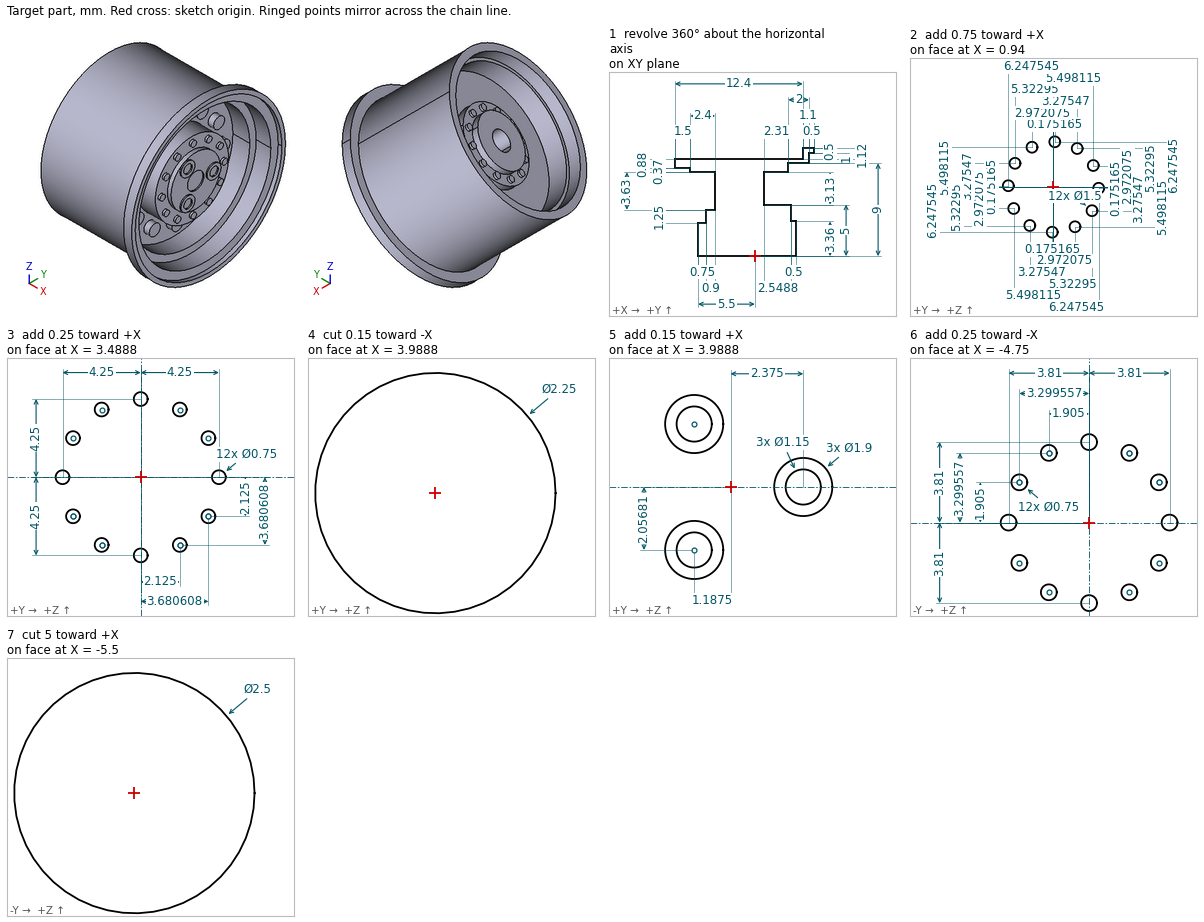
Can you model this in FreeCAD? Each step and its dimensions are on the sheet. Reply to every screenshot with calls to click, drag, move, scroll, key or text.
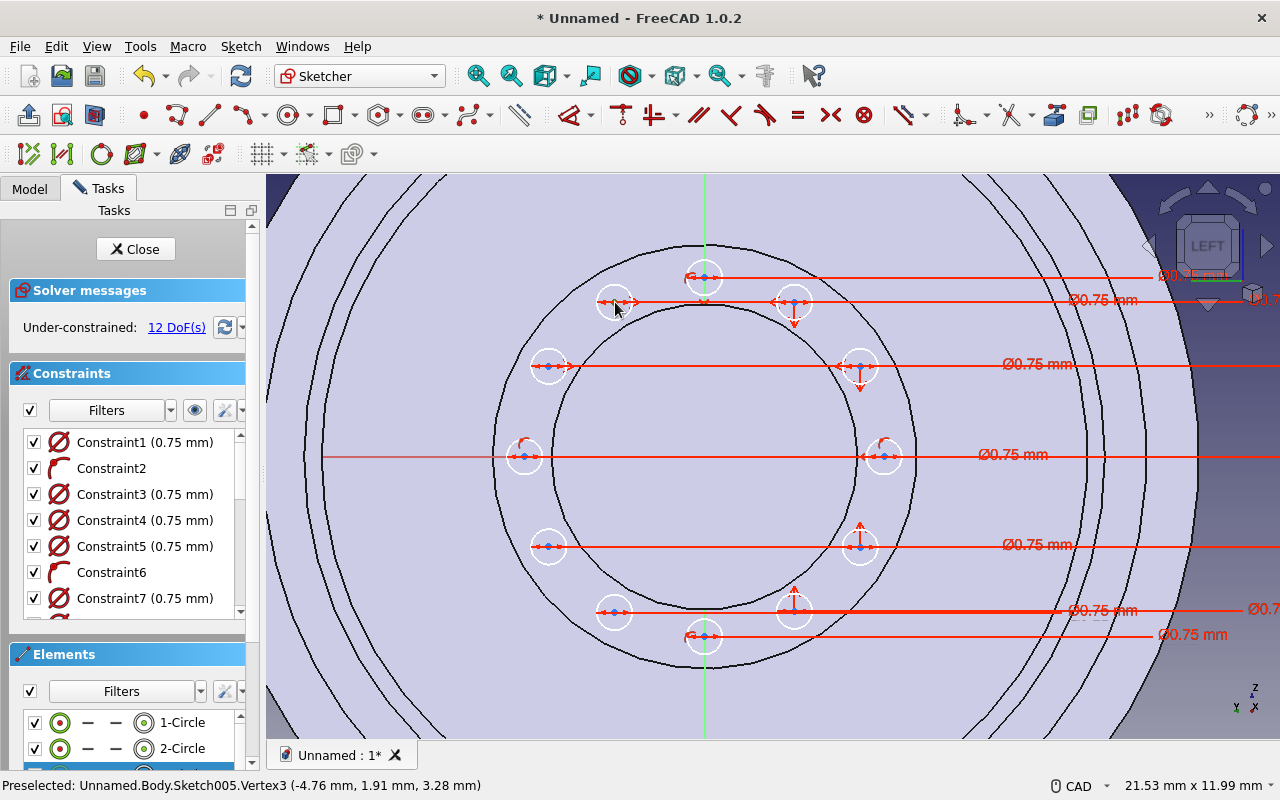
click(615, 613)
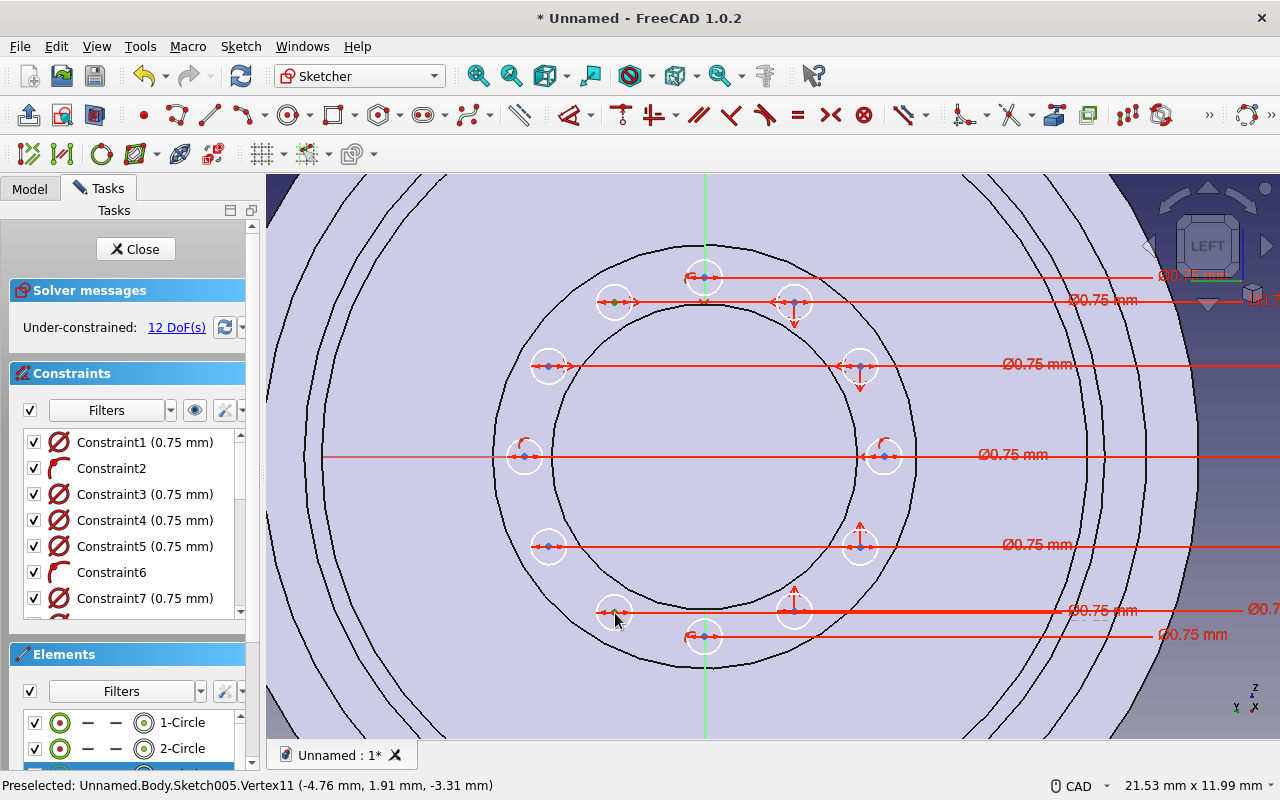
click(353, 457)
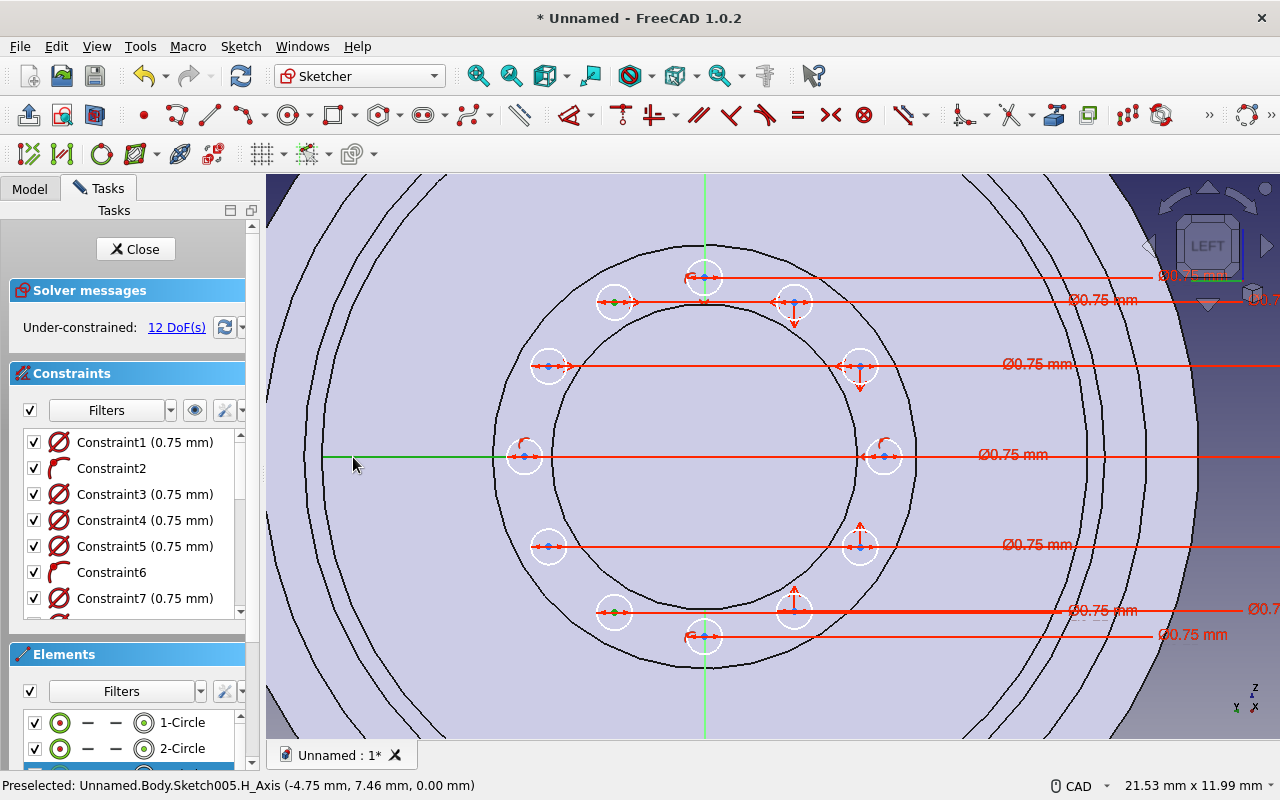
click(831, 116)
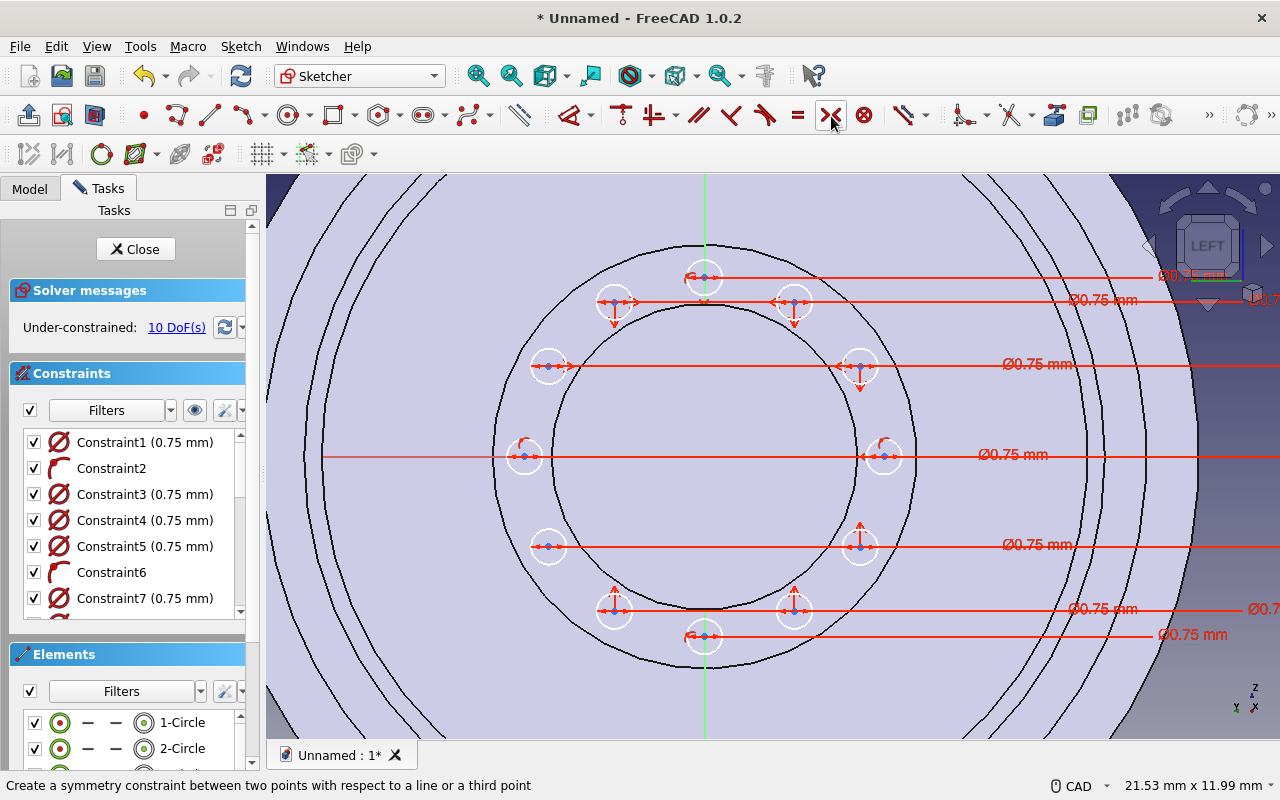
click(549, 366)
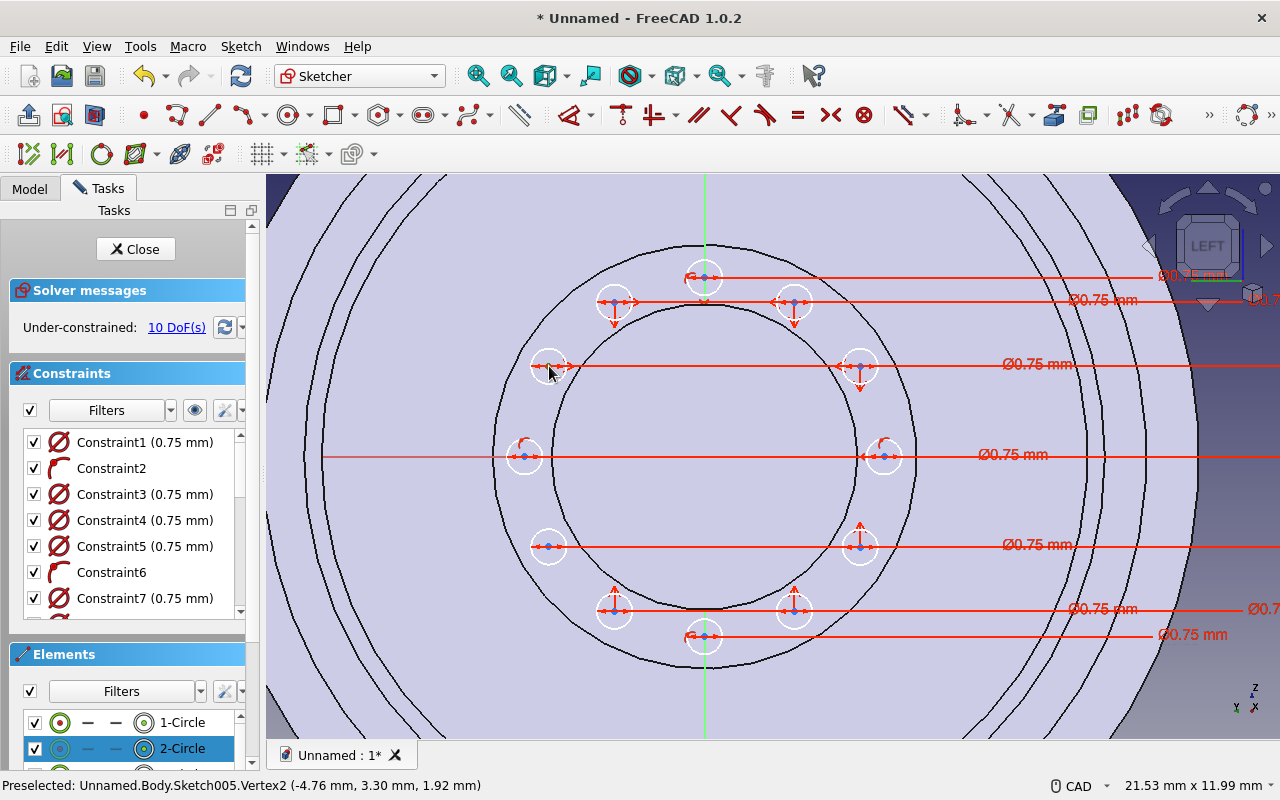
click(549, 547)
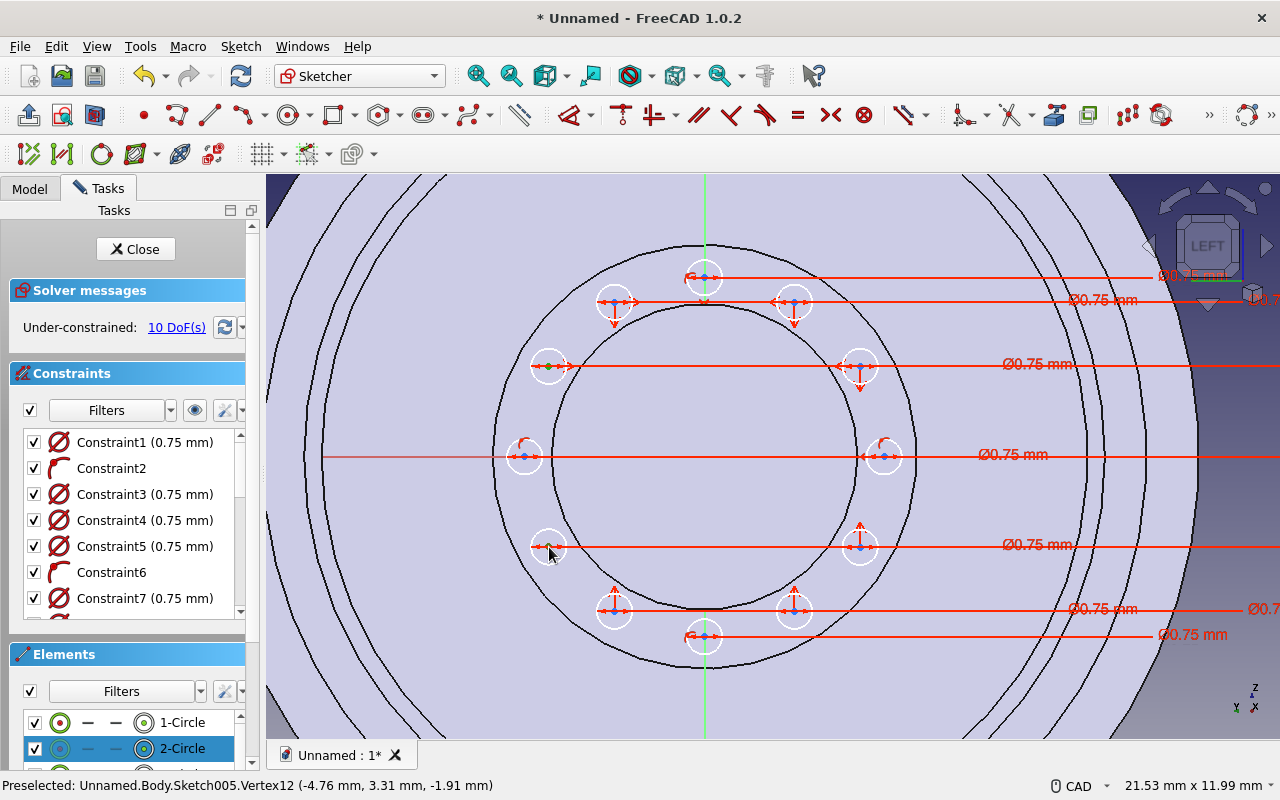
click(353, 457)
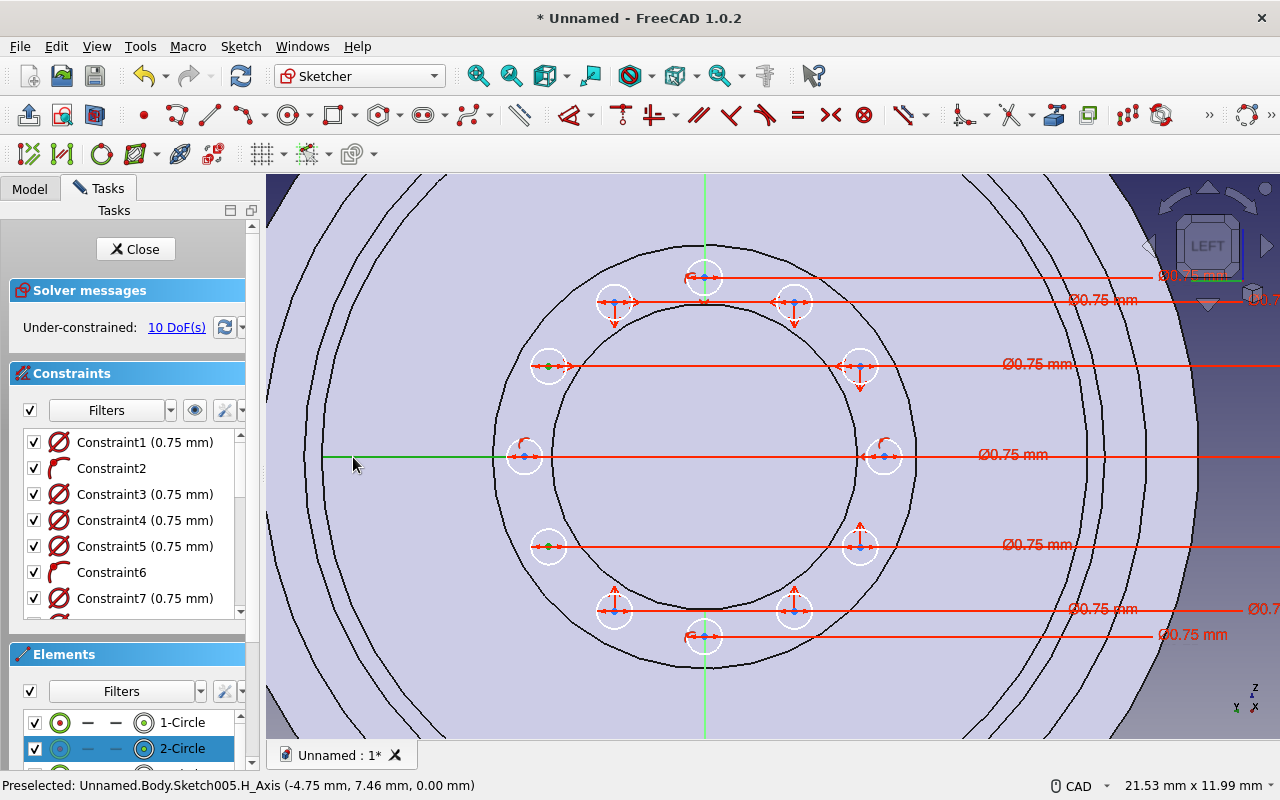
click(831, 116)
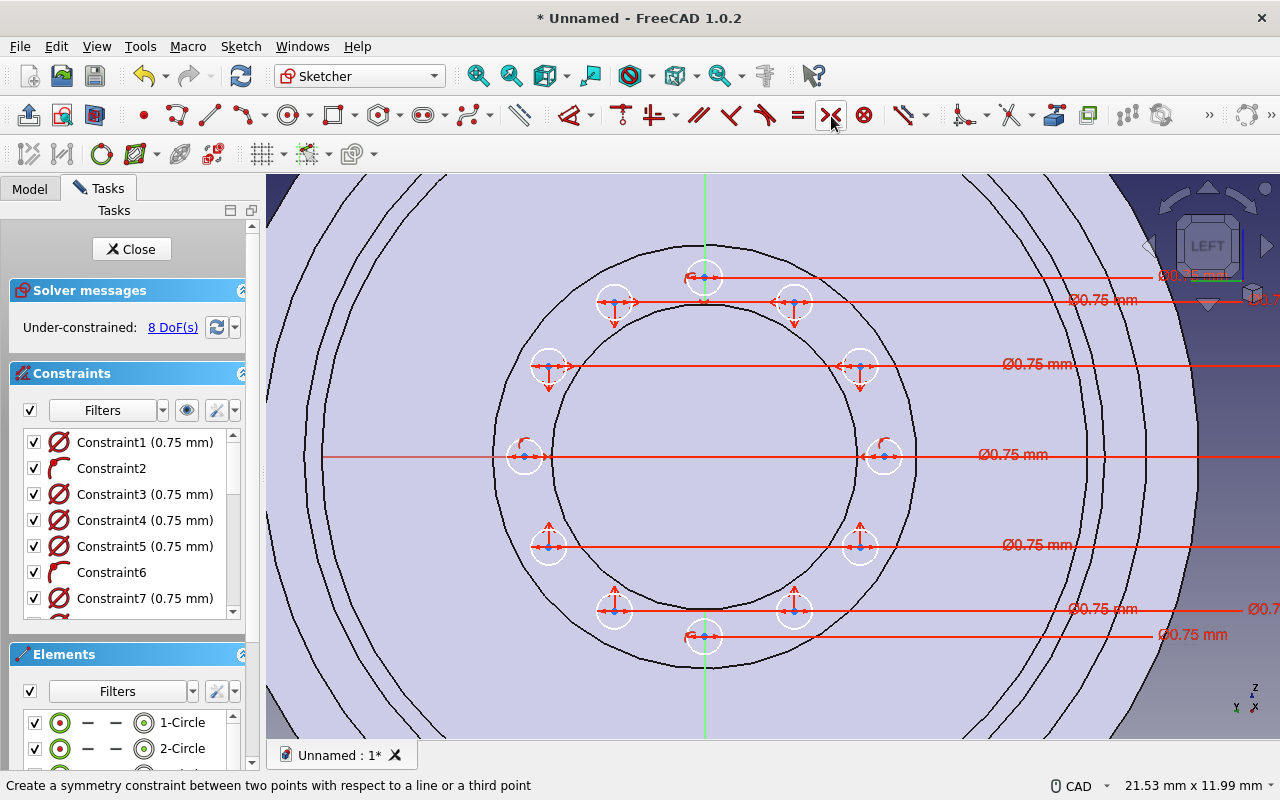
click(568, 116)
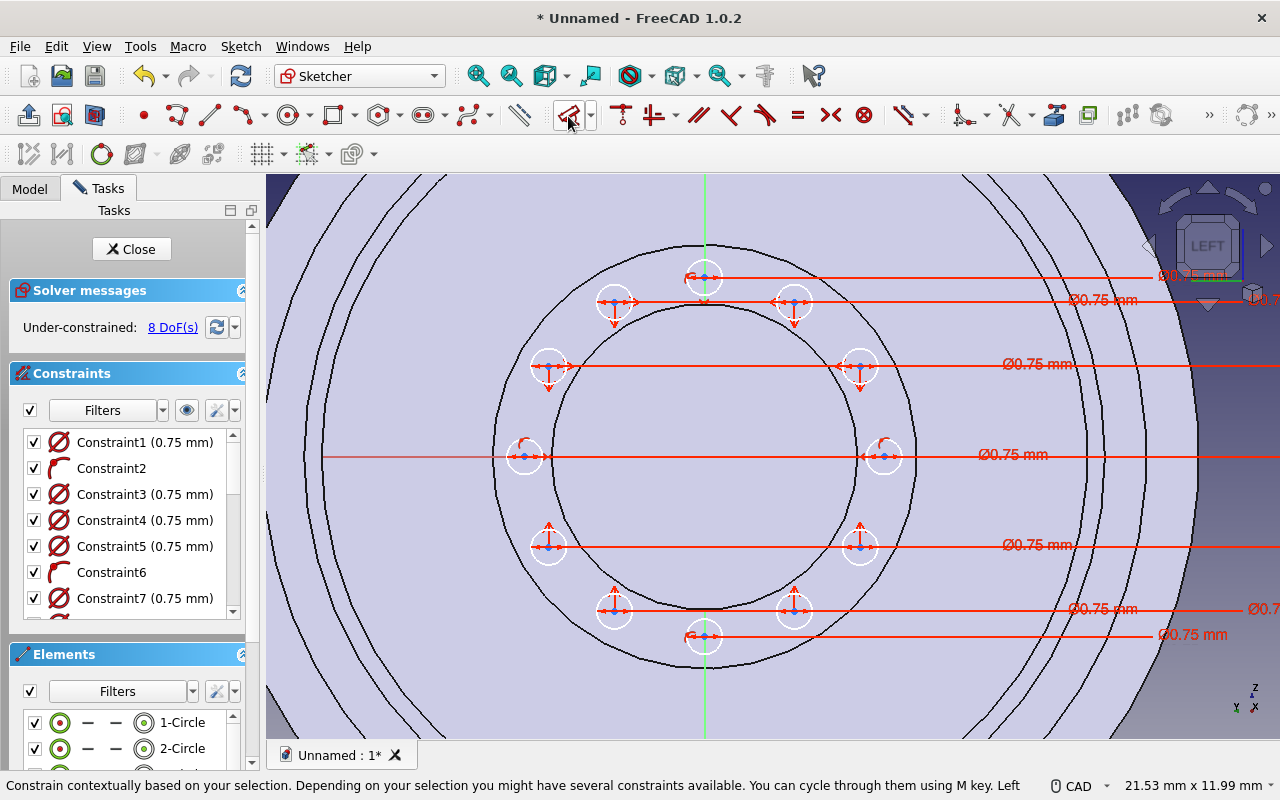
click(525, 457)
click(615, 491)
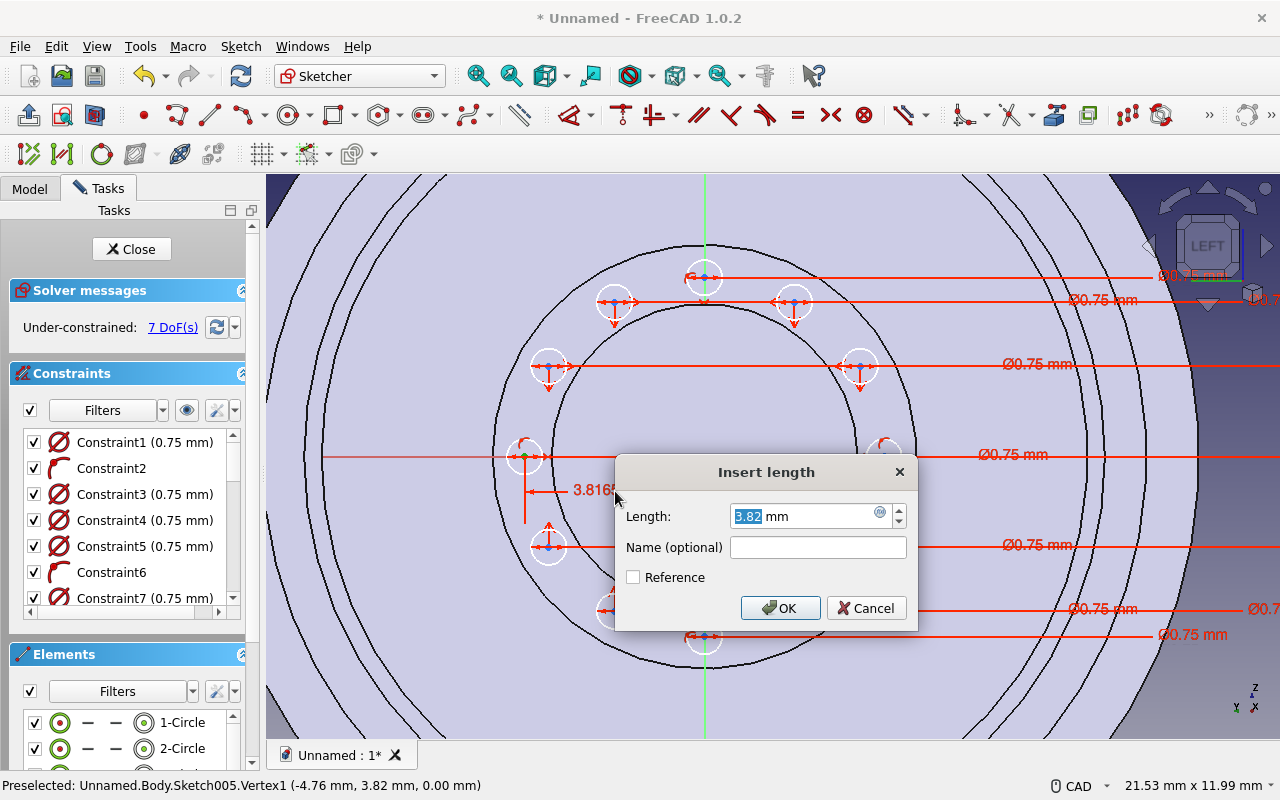
text(3.81)
key(Return)